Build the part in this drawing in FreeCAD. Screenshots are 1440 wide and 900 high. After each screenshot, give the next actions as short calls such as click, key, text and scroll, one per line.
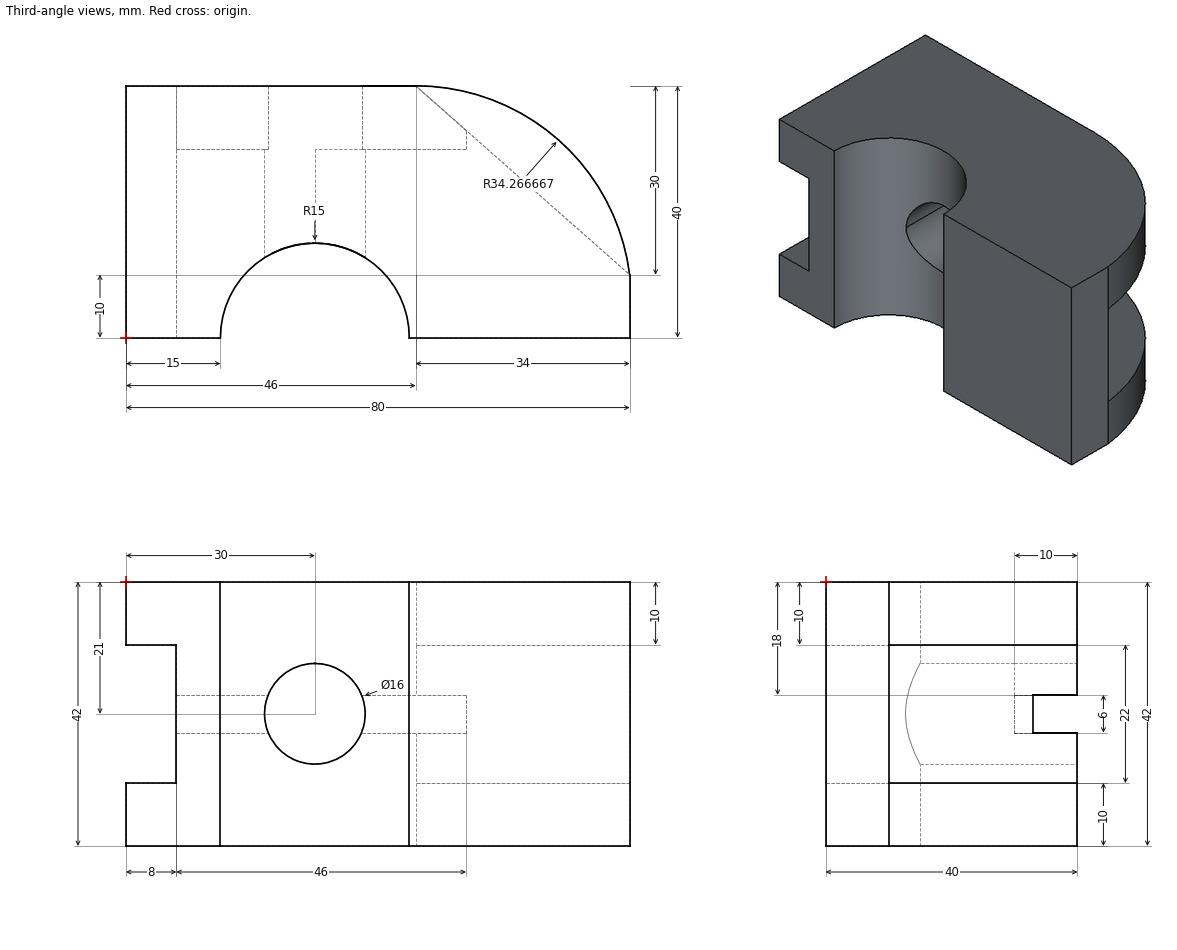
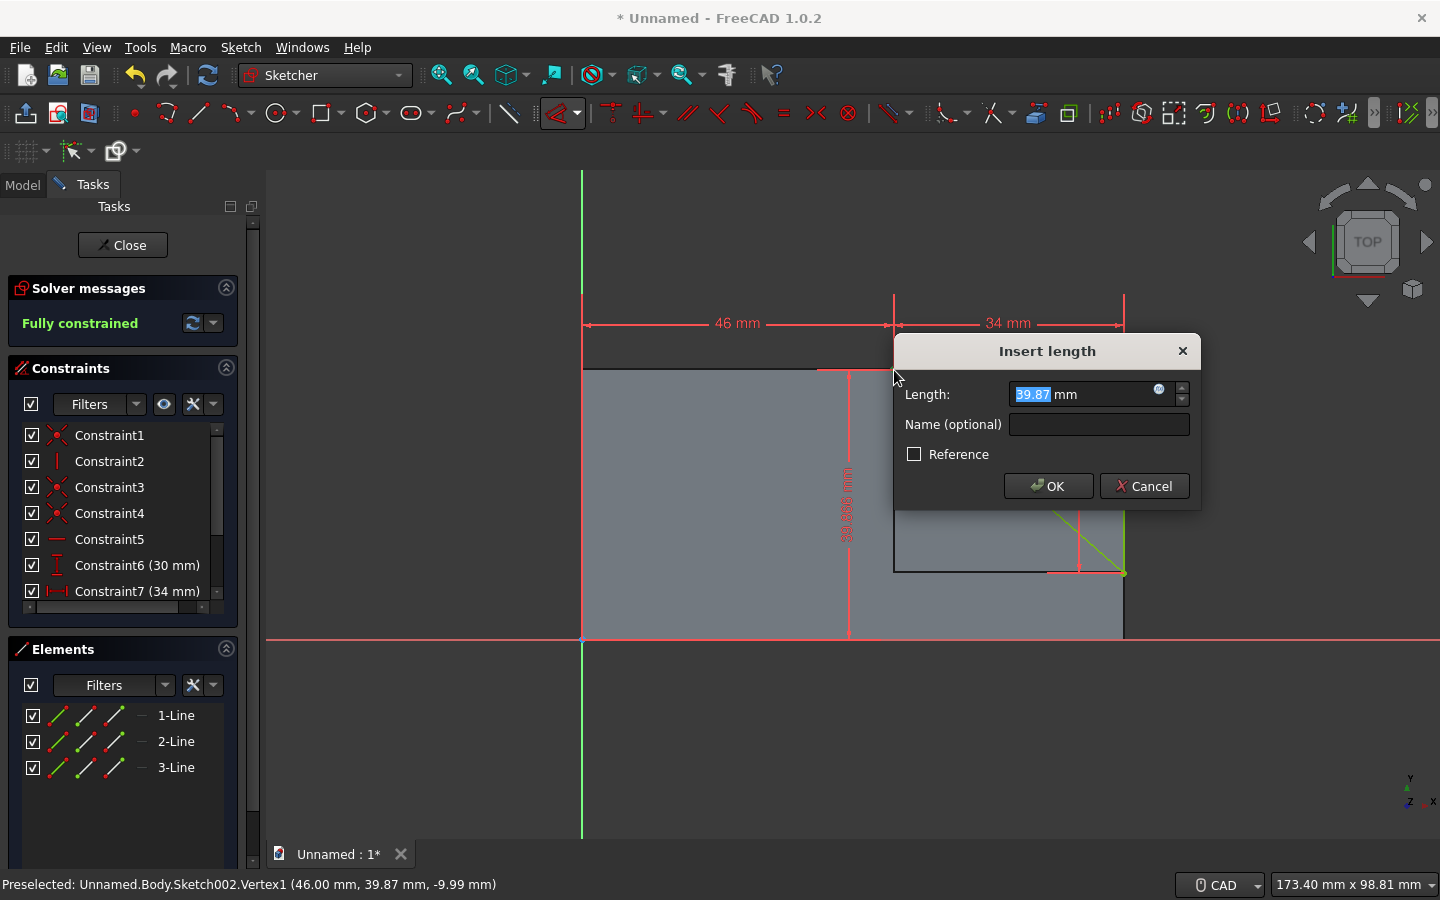
text(40)
key(Return)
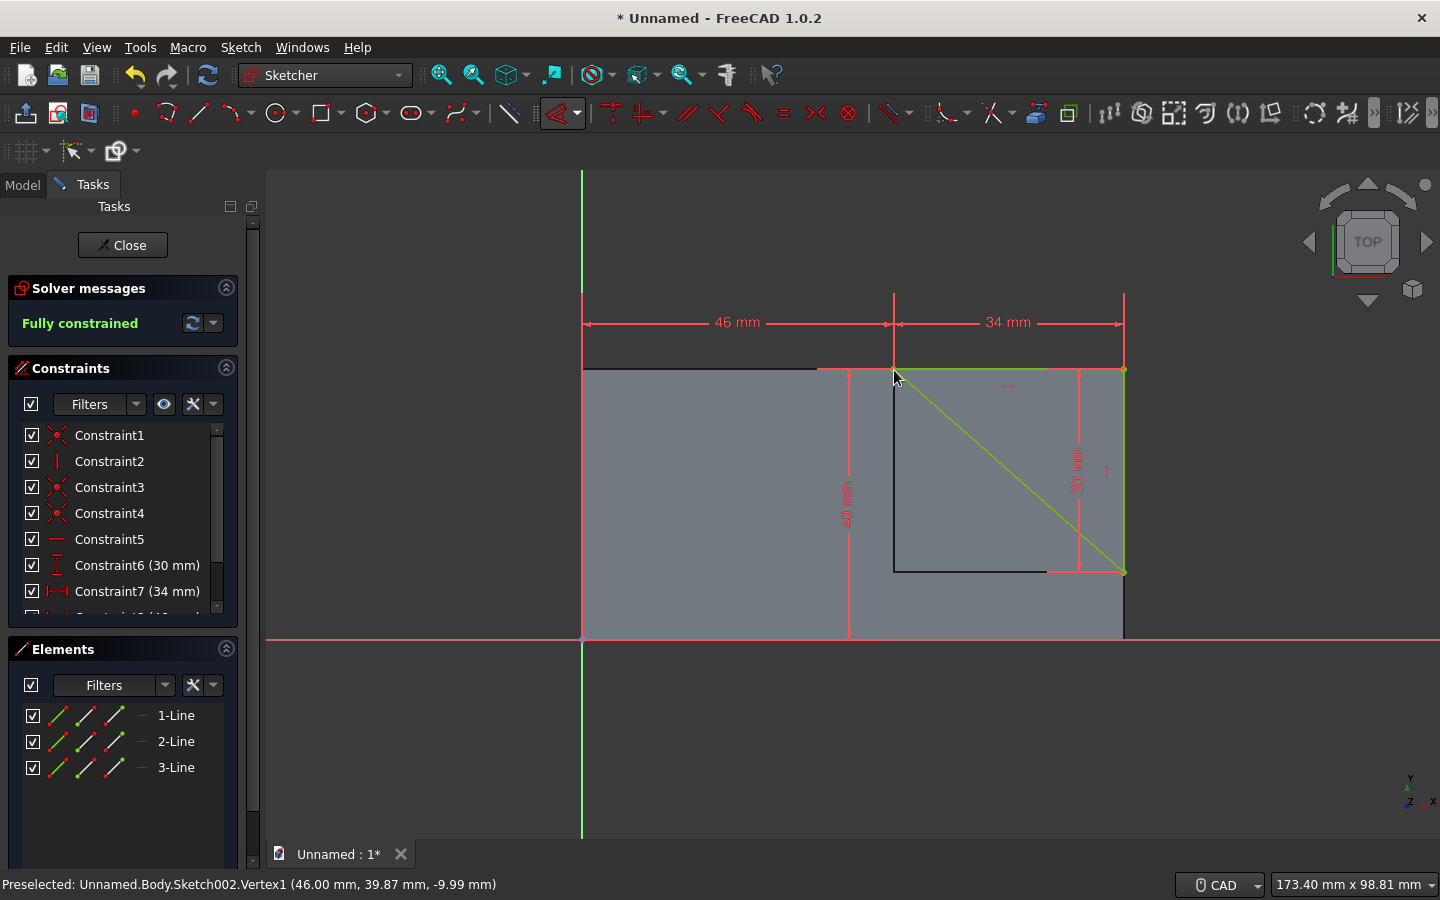
click(123, 245)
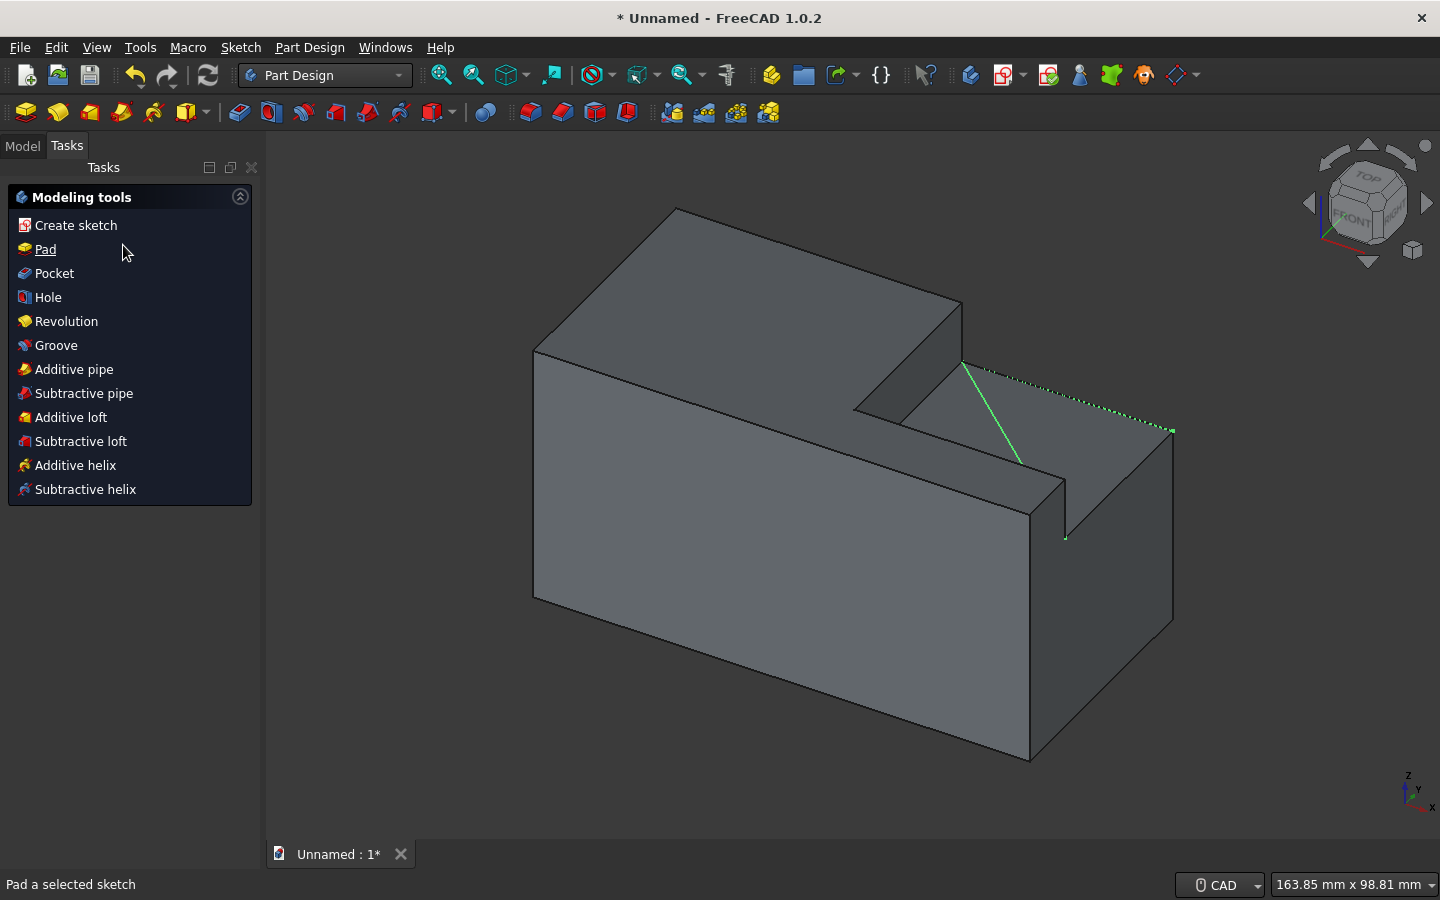
click(240, 112)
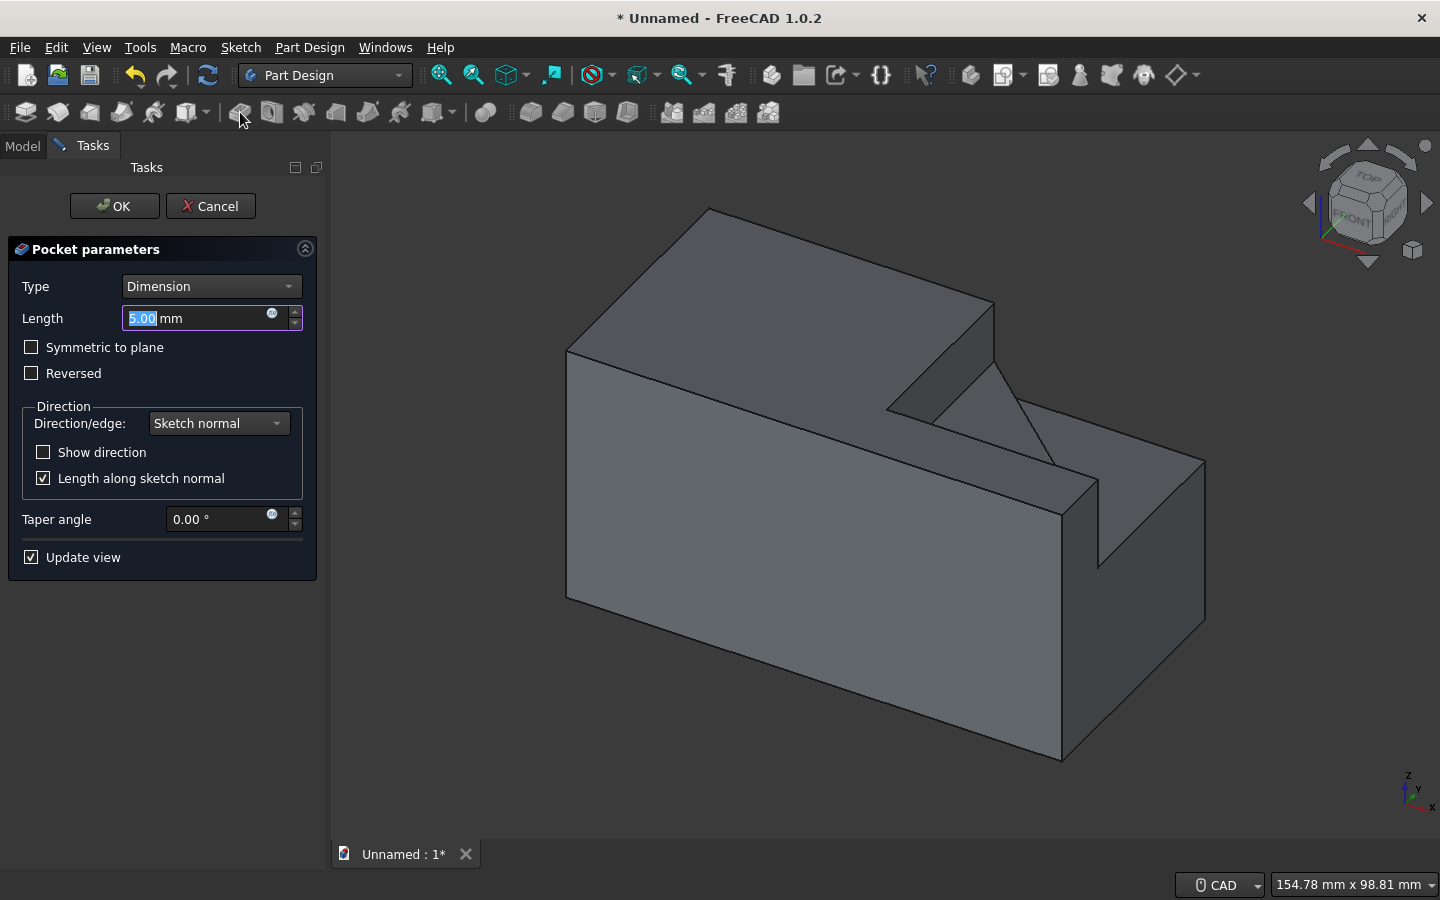
text(22)
key(Tab)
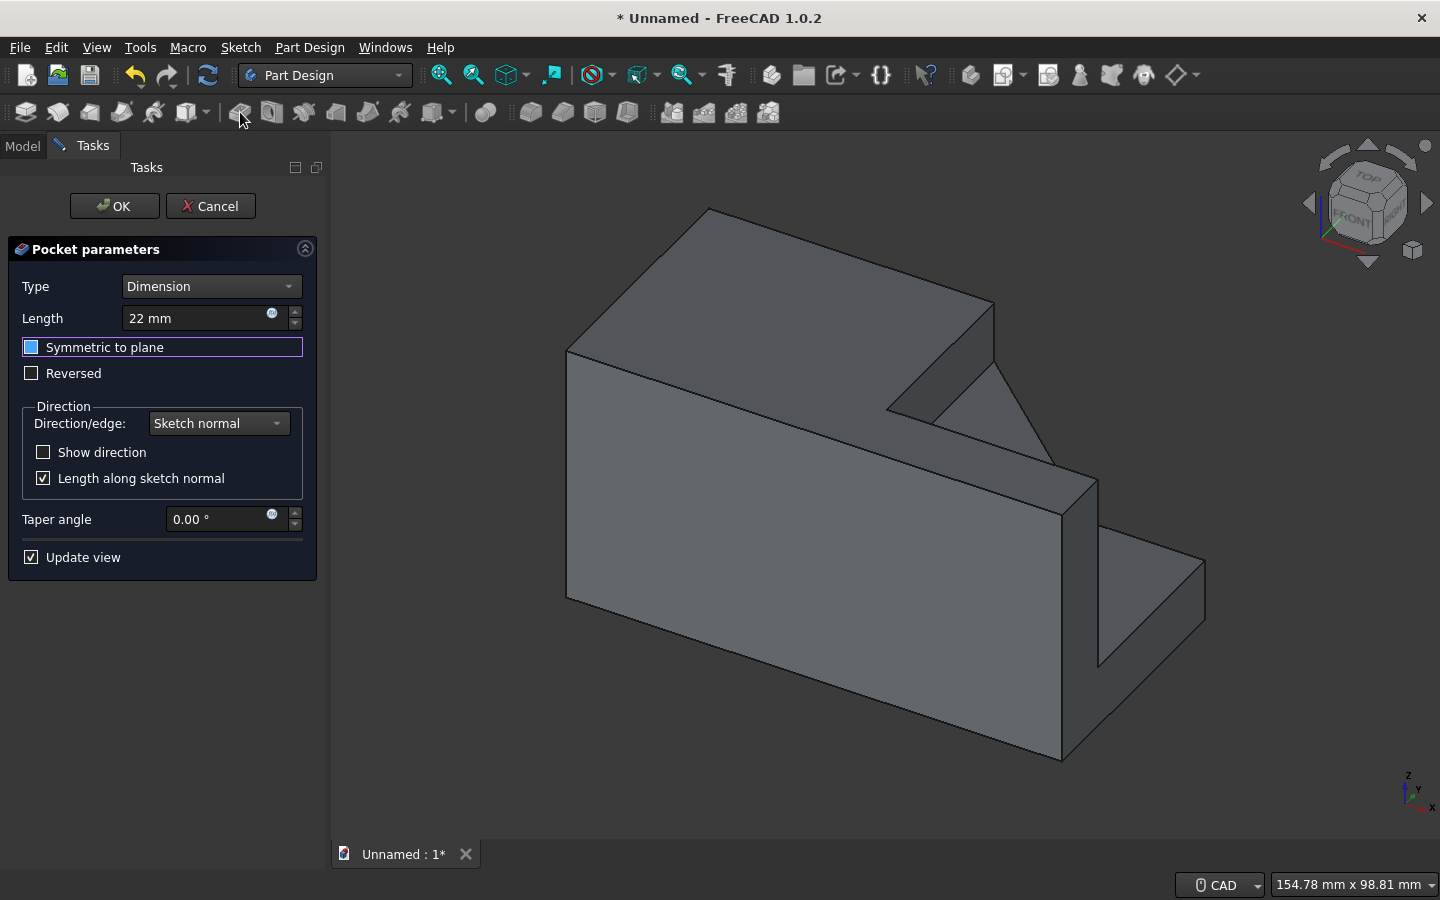
click(115, 206)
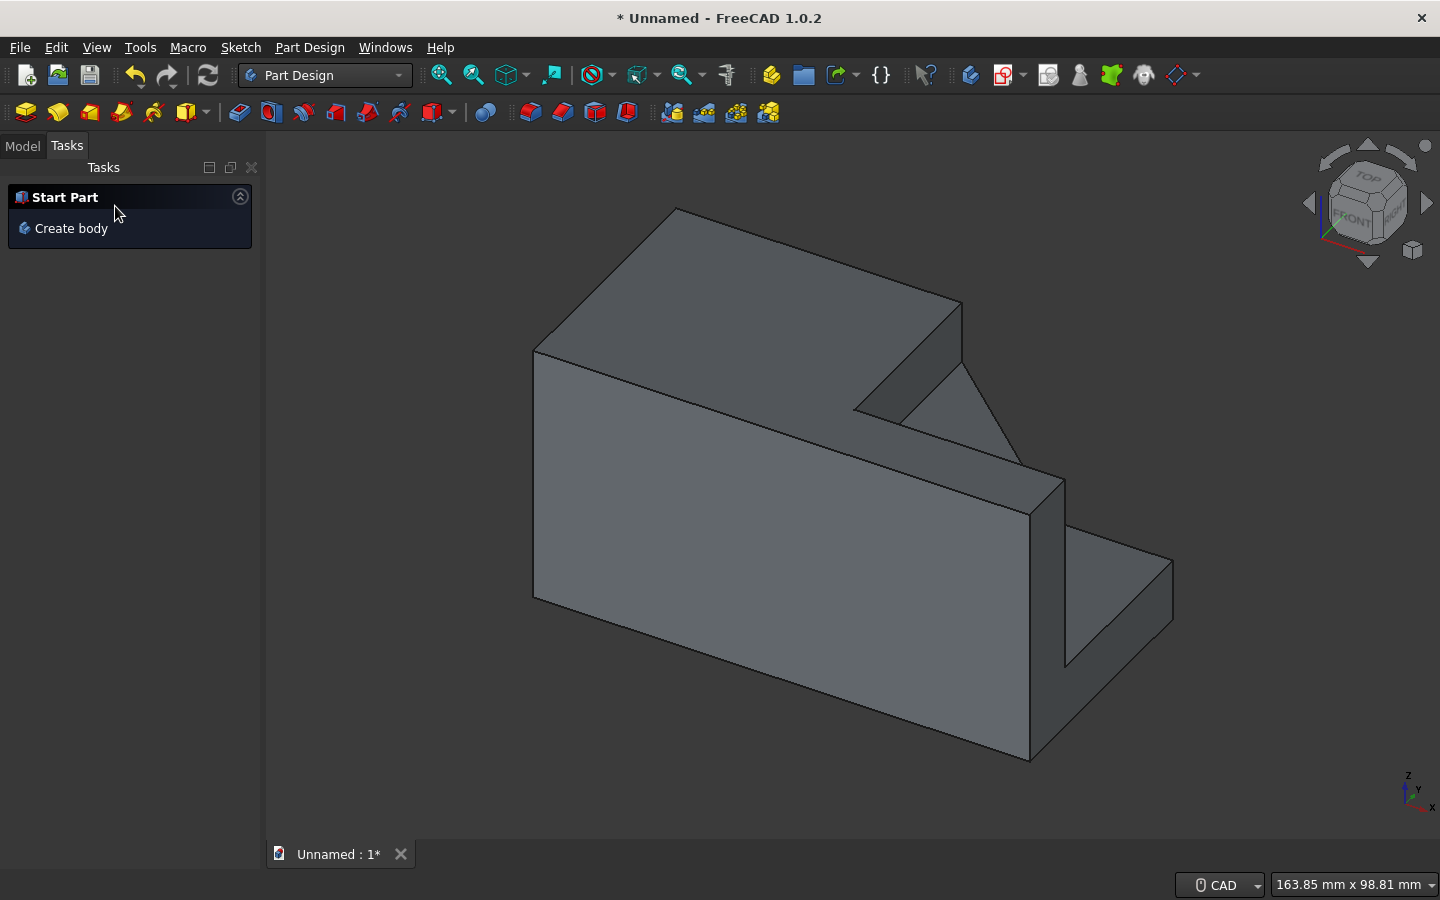
click(1004, 76)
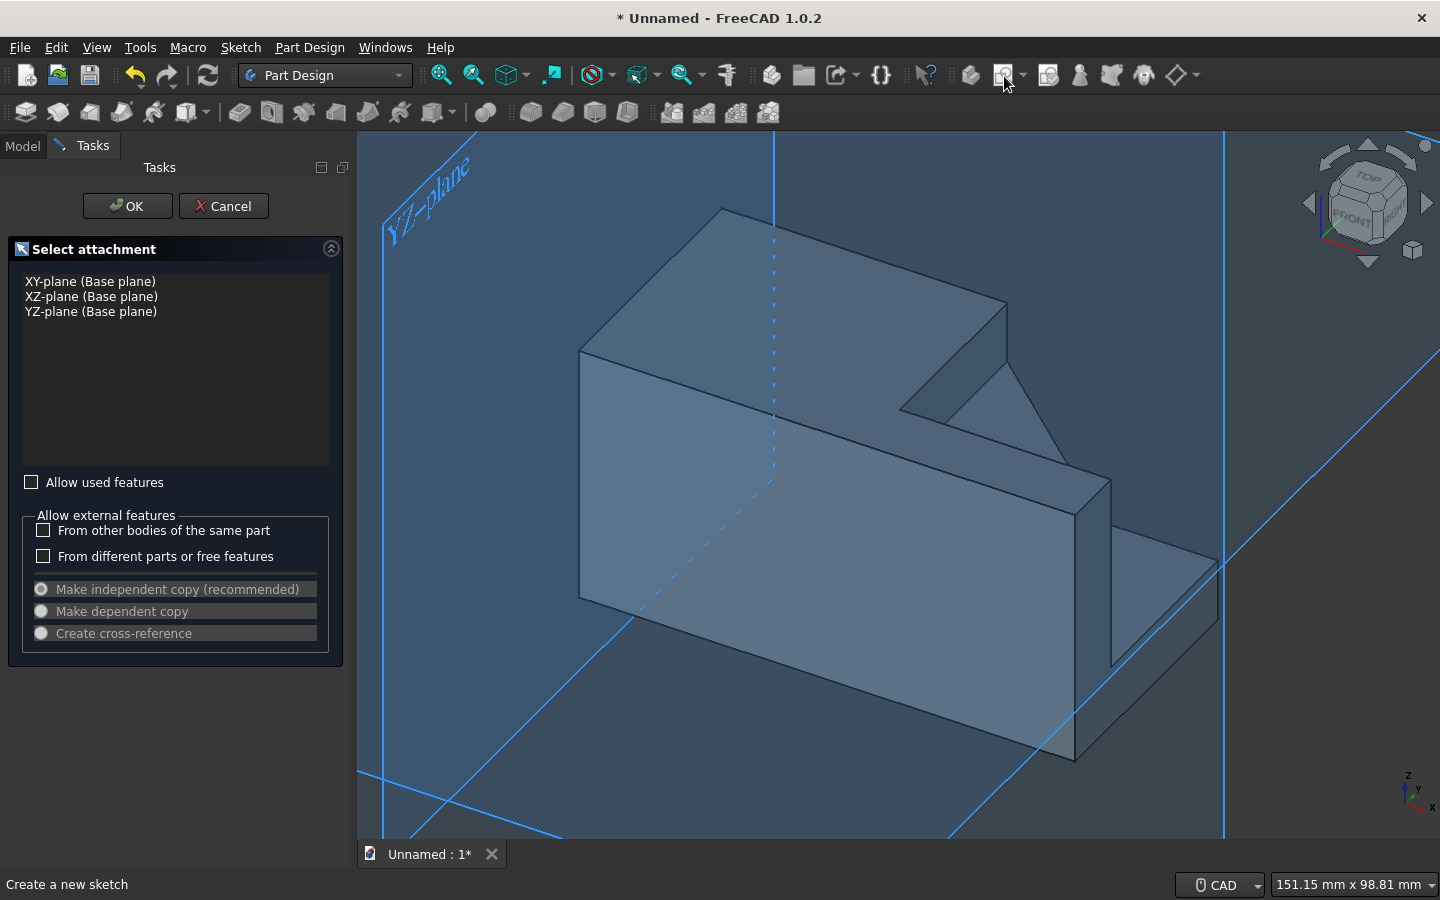
click(82, 282)